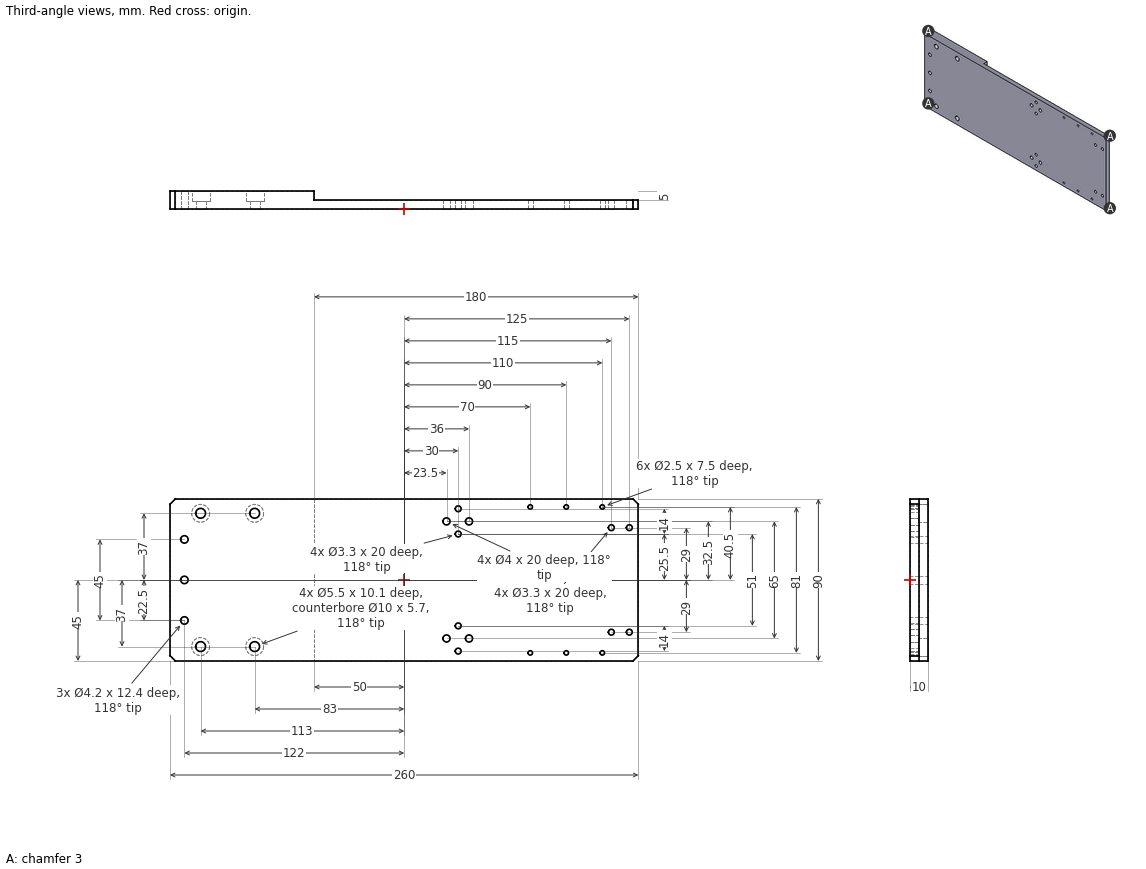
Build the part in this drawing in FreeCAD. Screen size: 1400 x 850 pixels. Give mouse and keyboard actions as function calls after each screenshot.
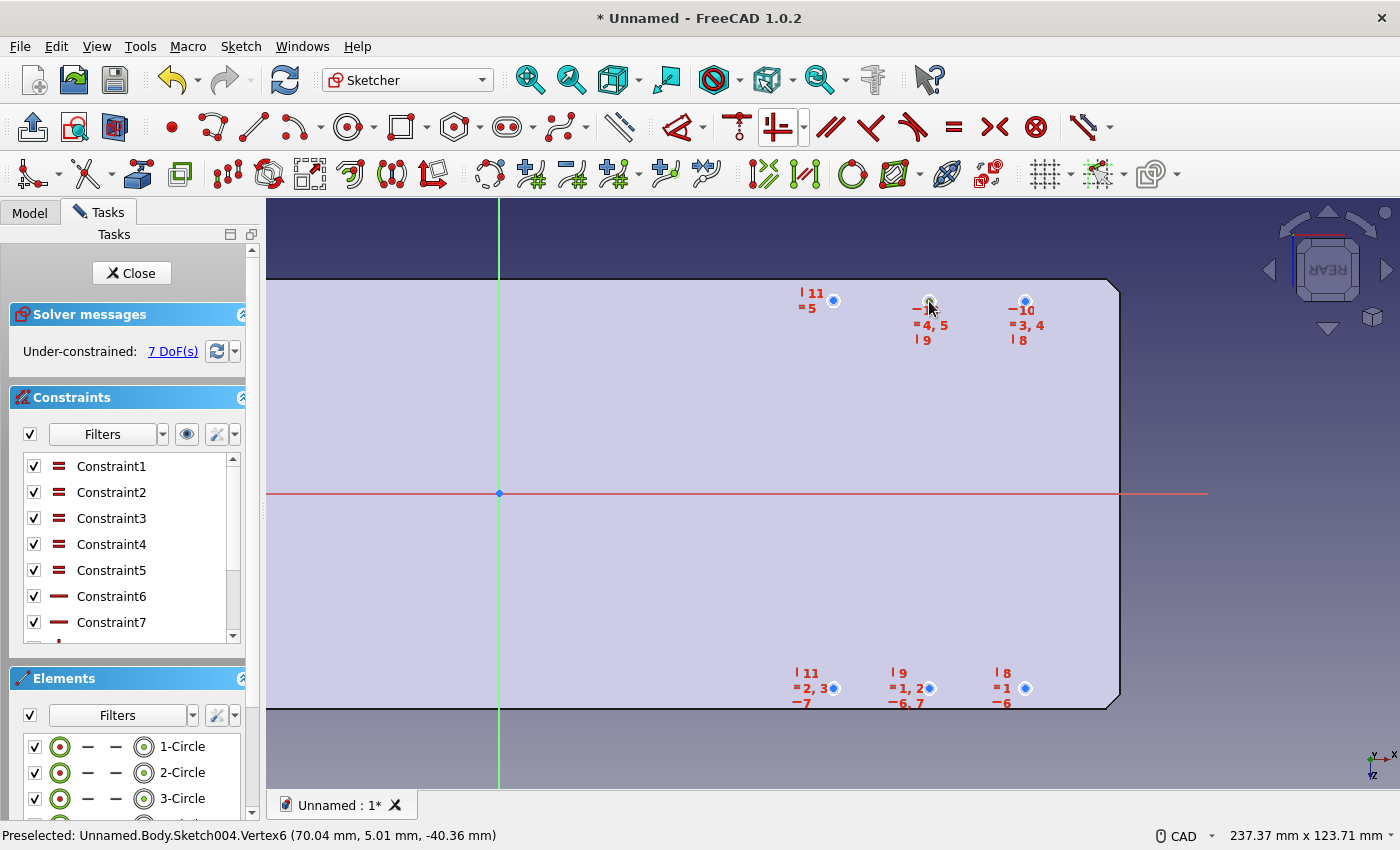
click(834, 301)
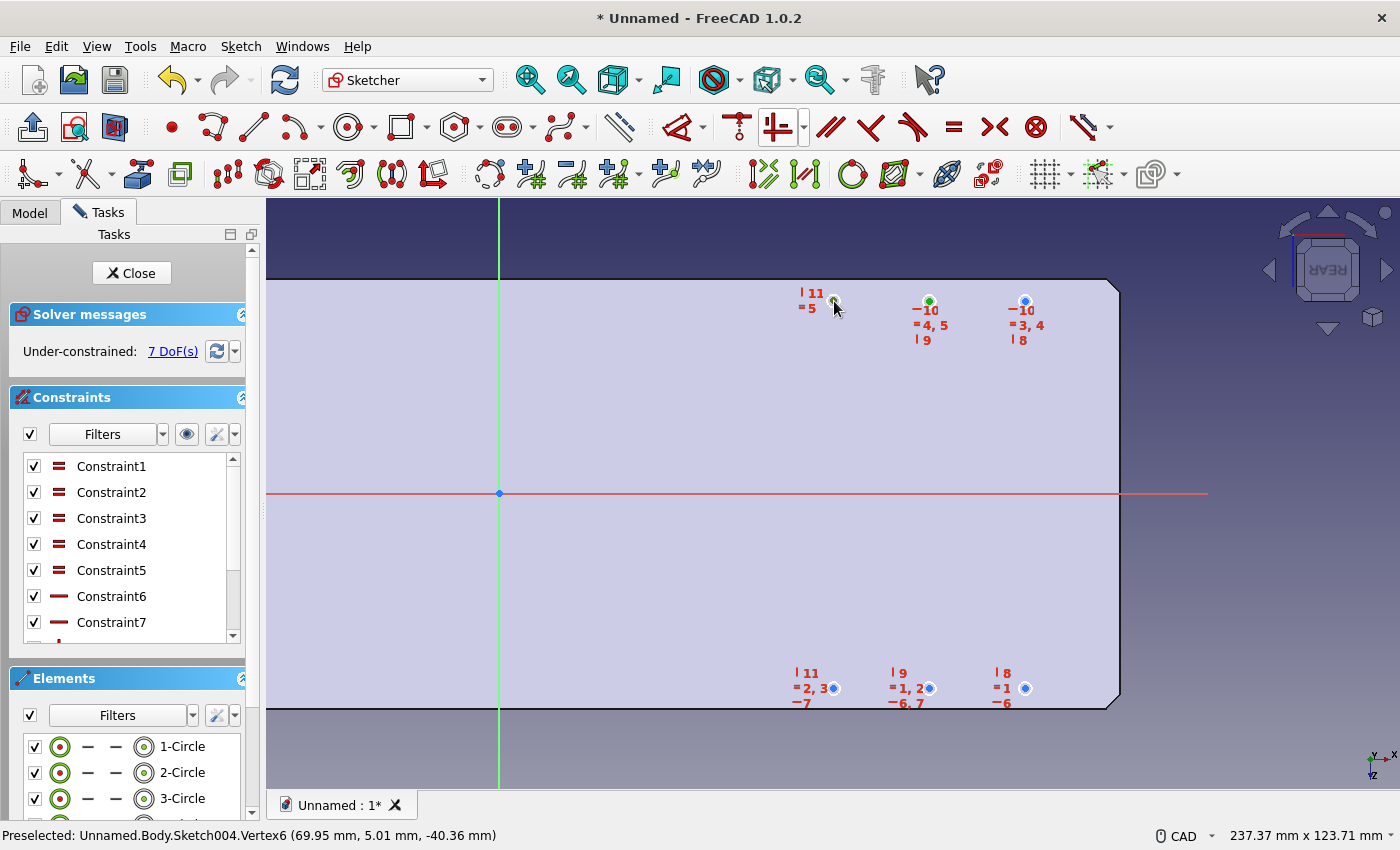
click(804, 128)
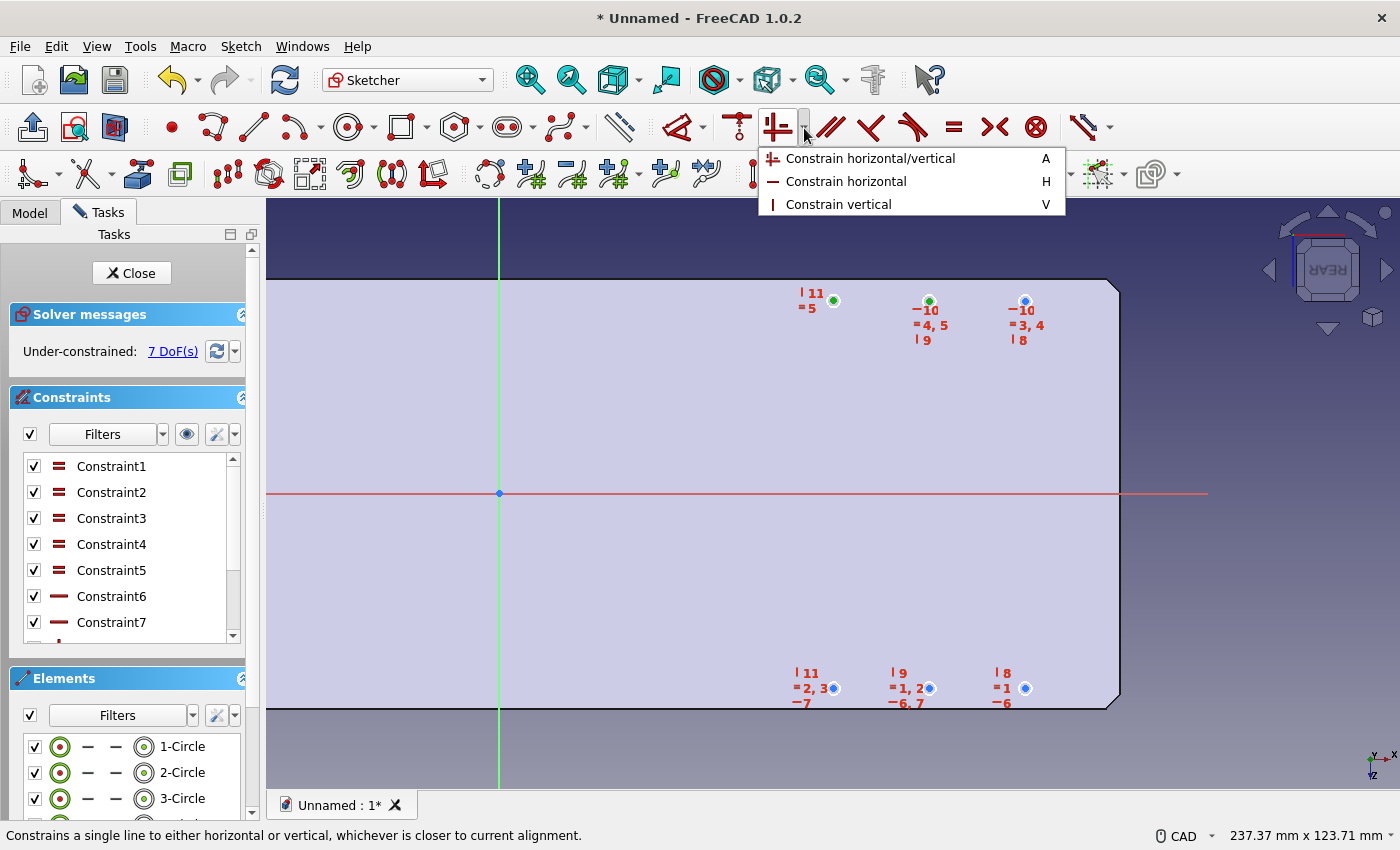
click(912, 182)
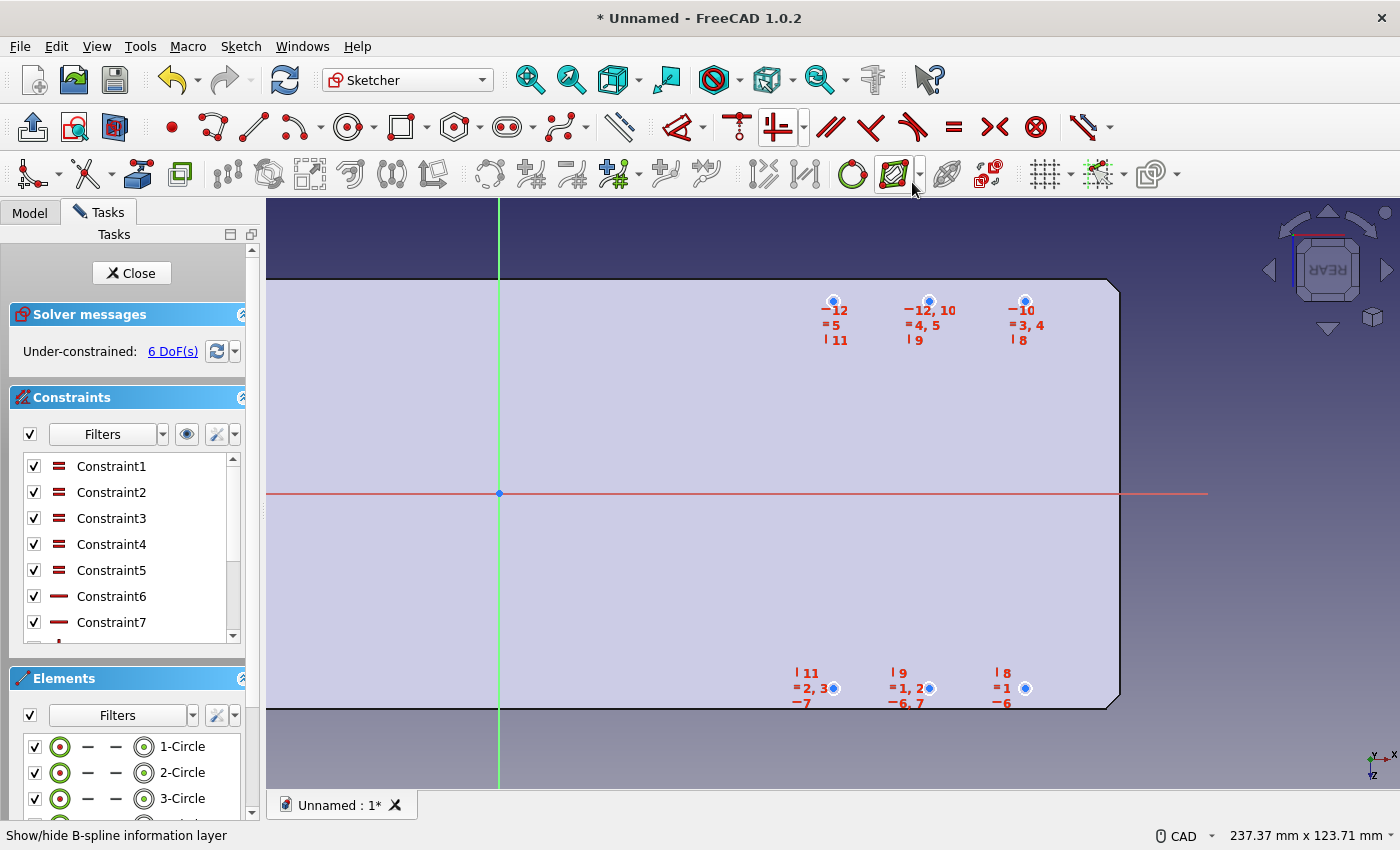
click(676, 128)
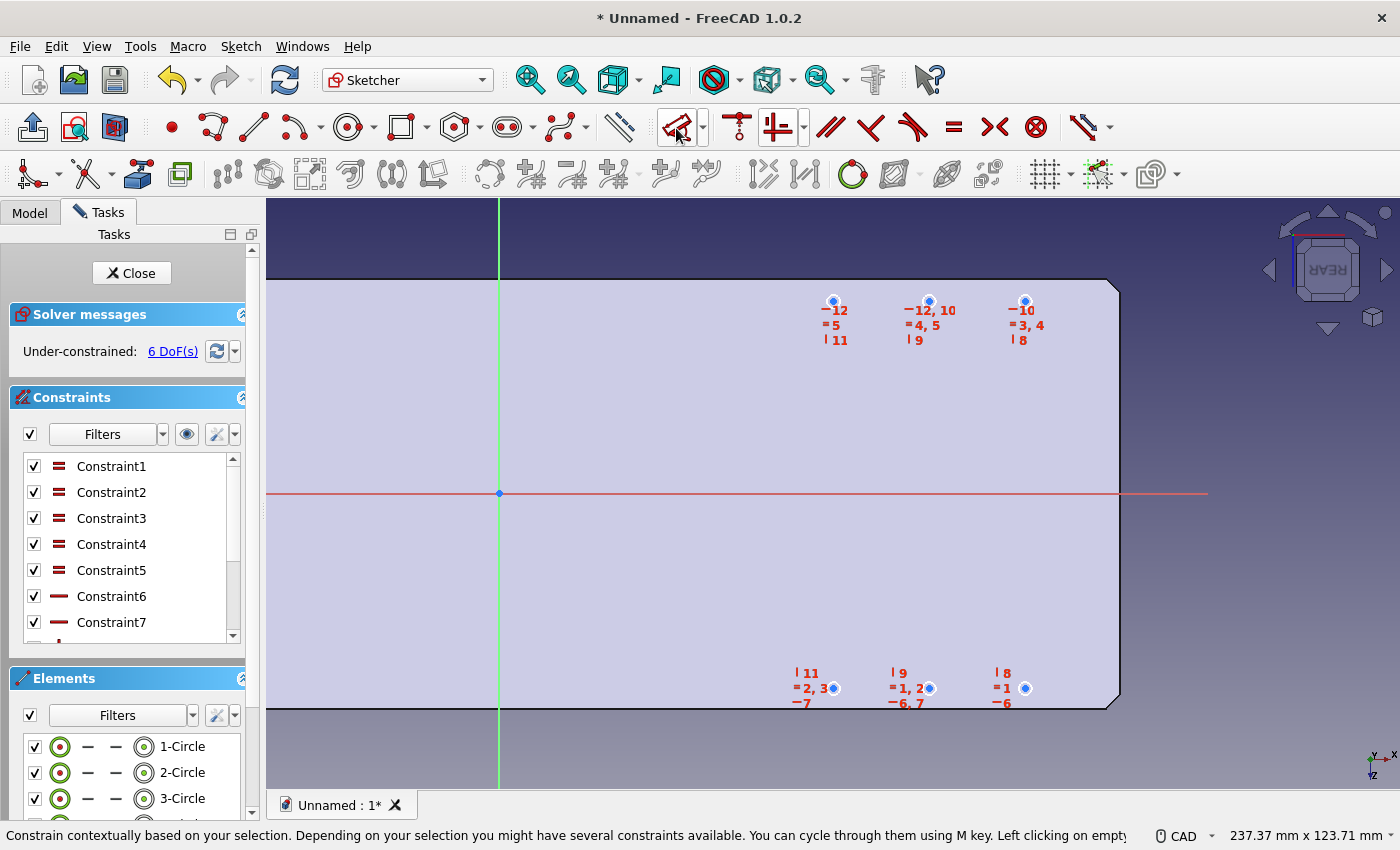
scroll(1019, 688, up, 7)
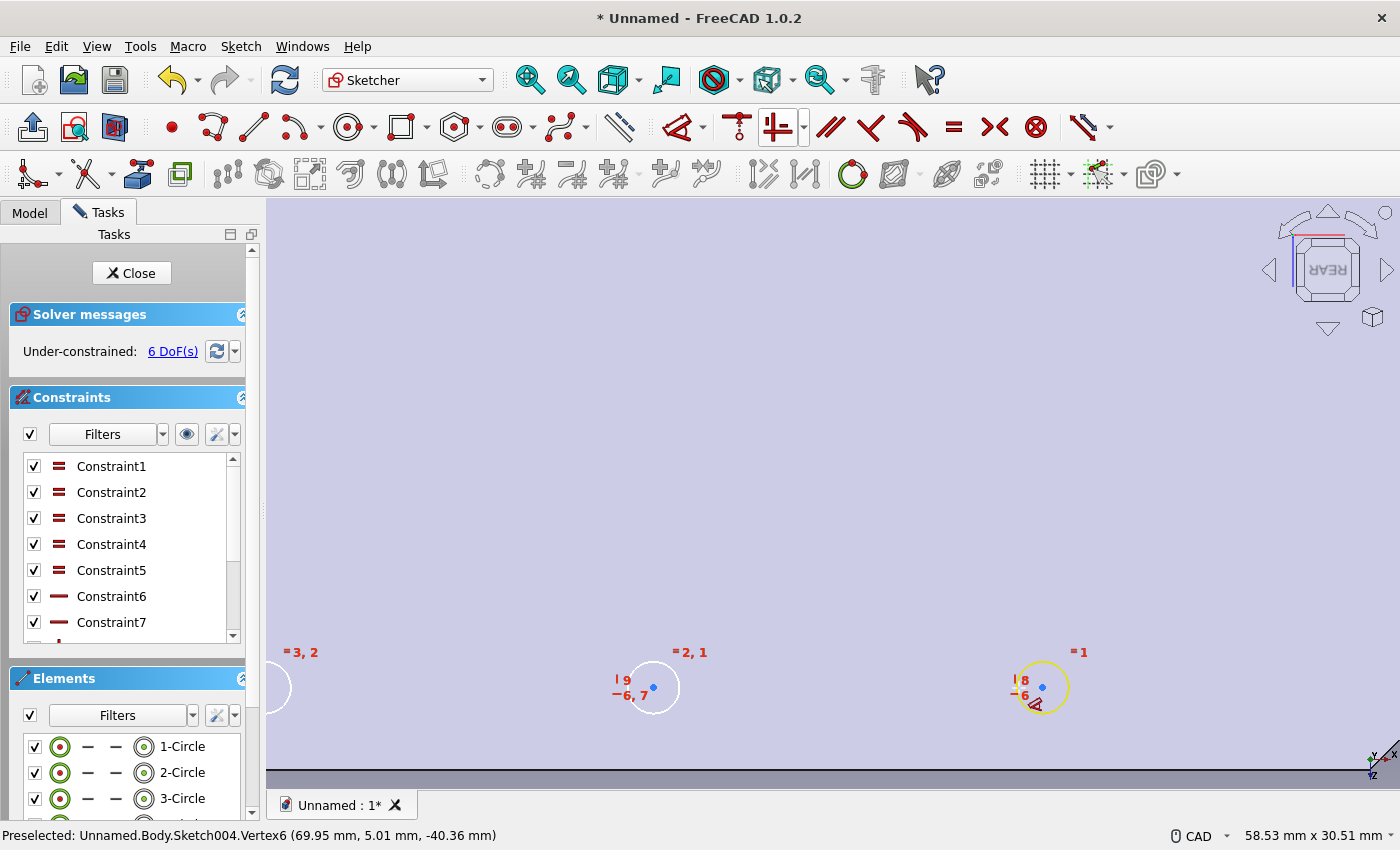
click(1017, 687)
click(985, 686)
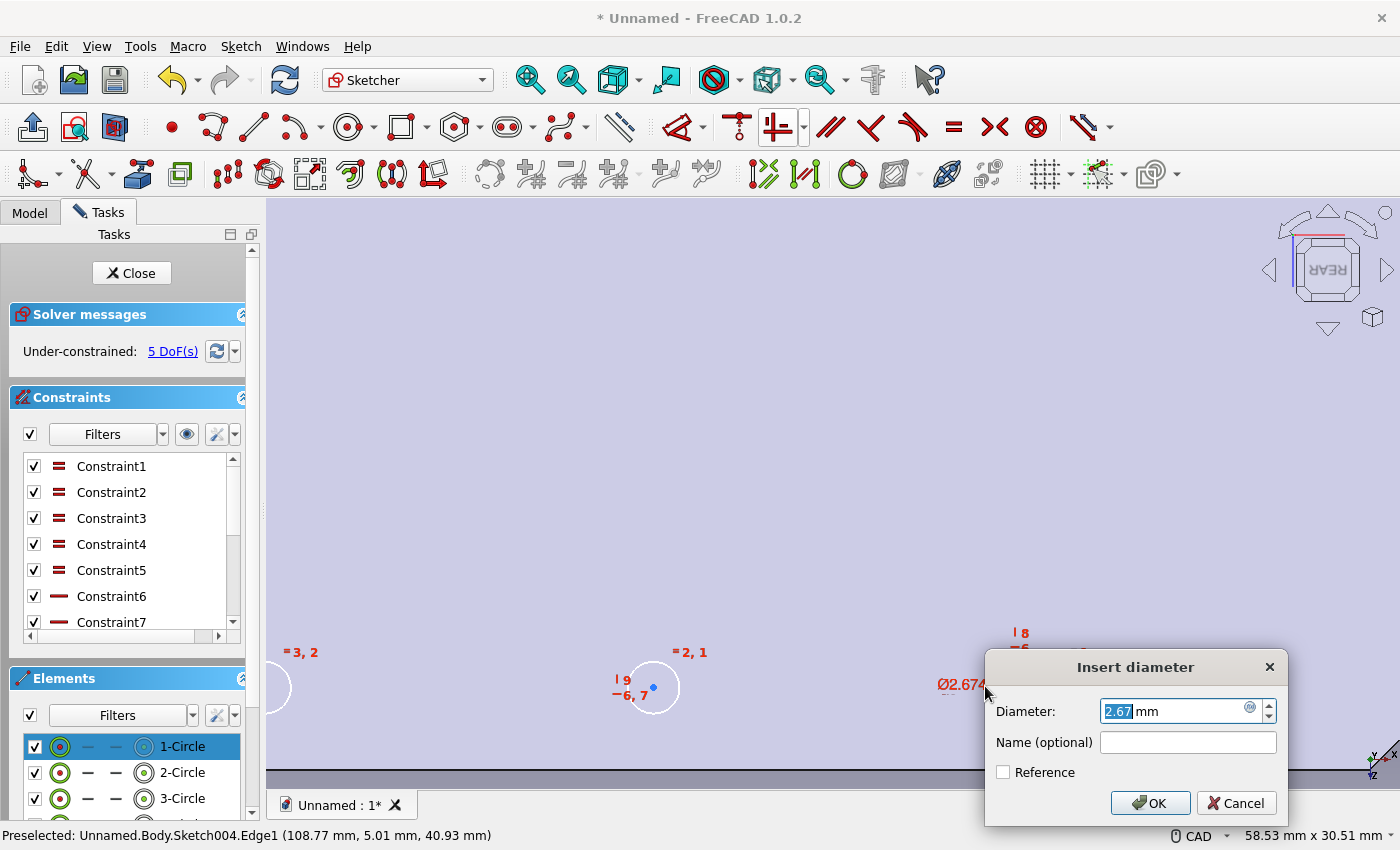
text(2.5)
key(Return)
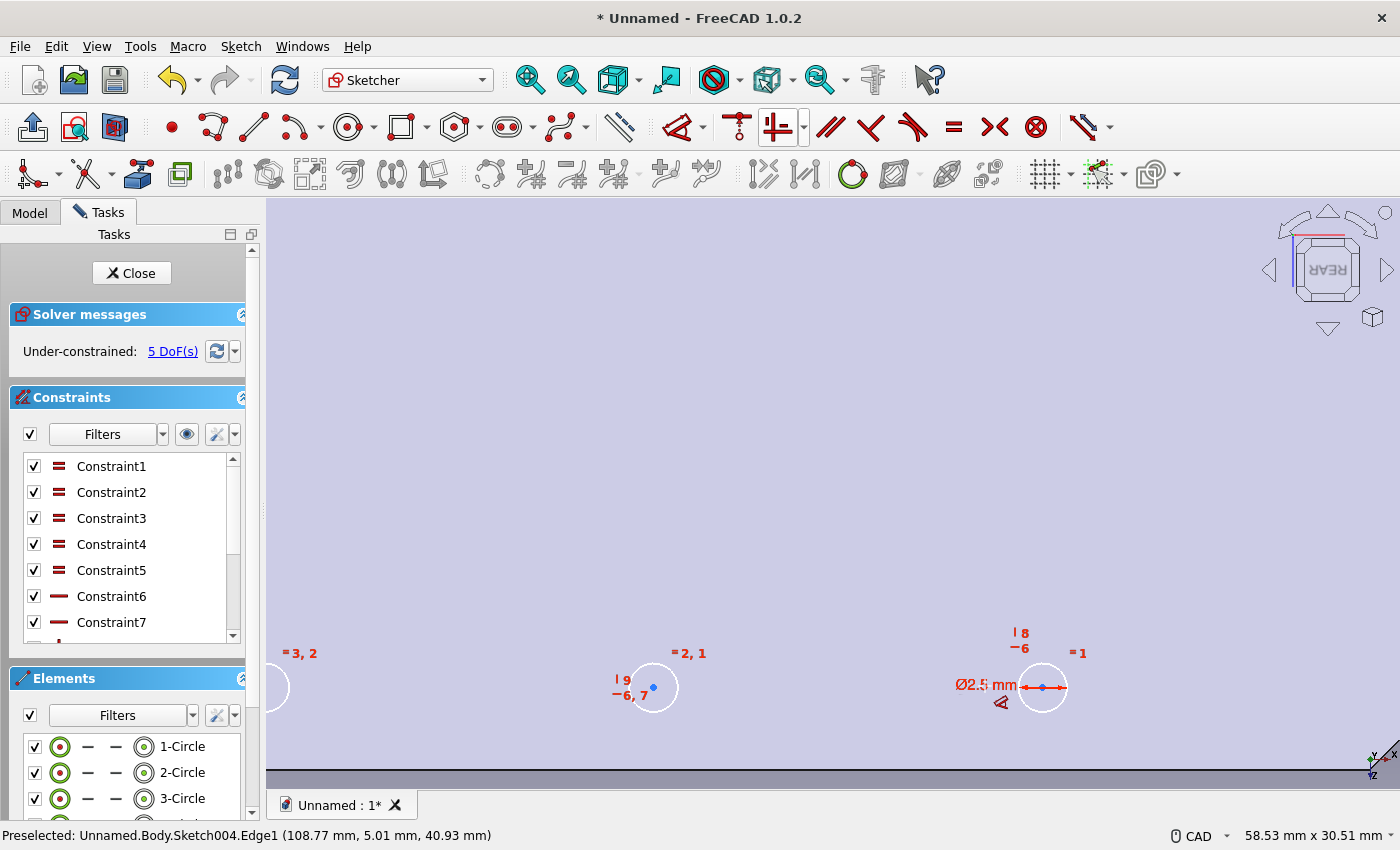
scroll(1019, 688, down, 7)